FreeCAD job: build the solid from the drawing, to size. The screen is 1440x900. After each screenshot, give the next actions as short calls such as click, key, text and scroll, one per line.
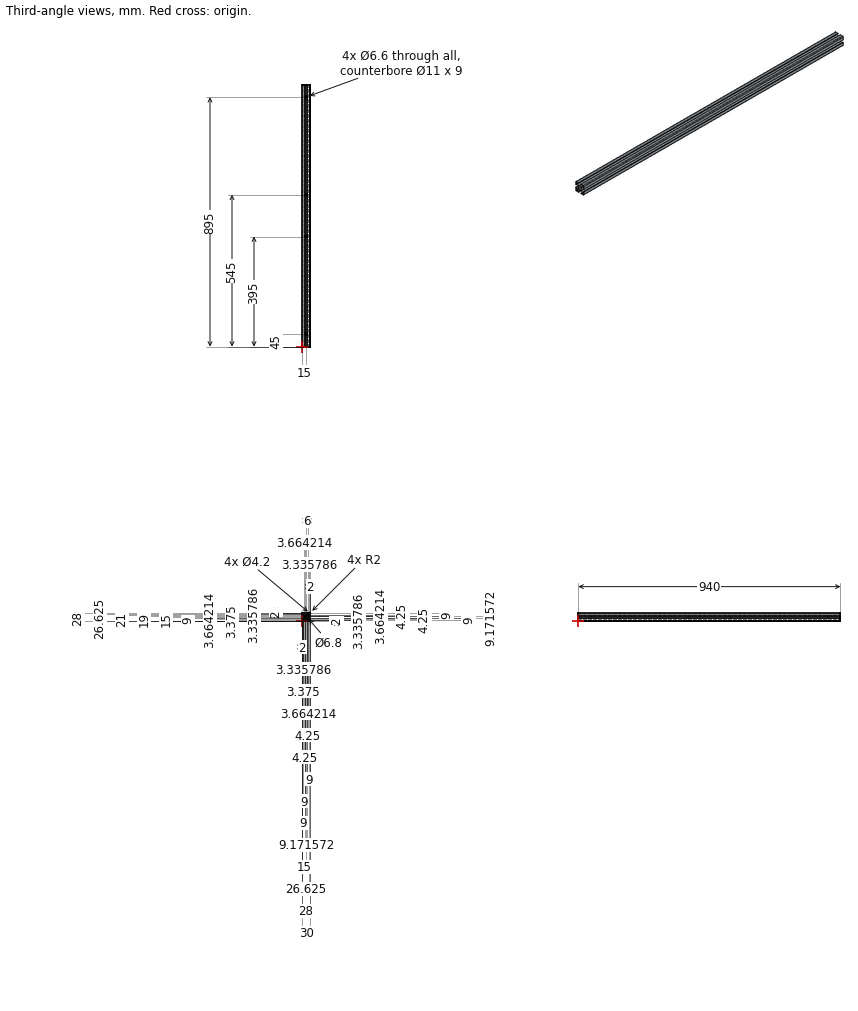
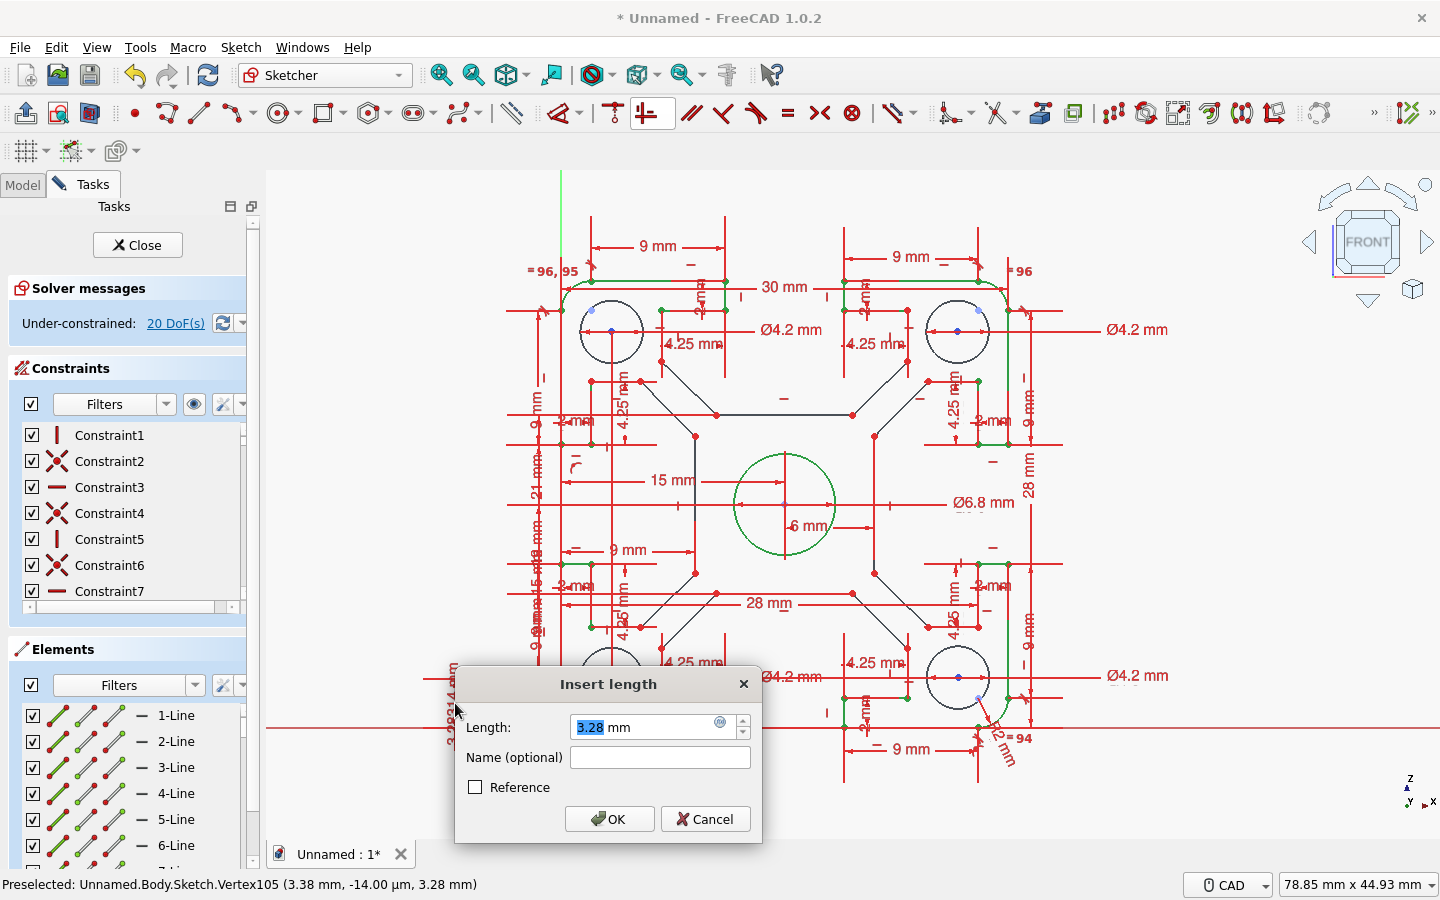
text(3.375)
key(Return)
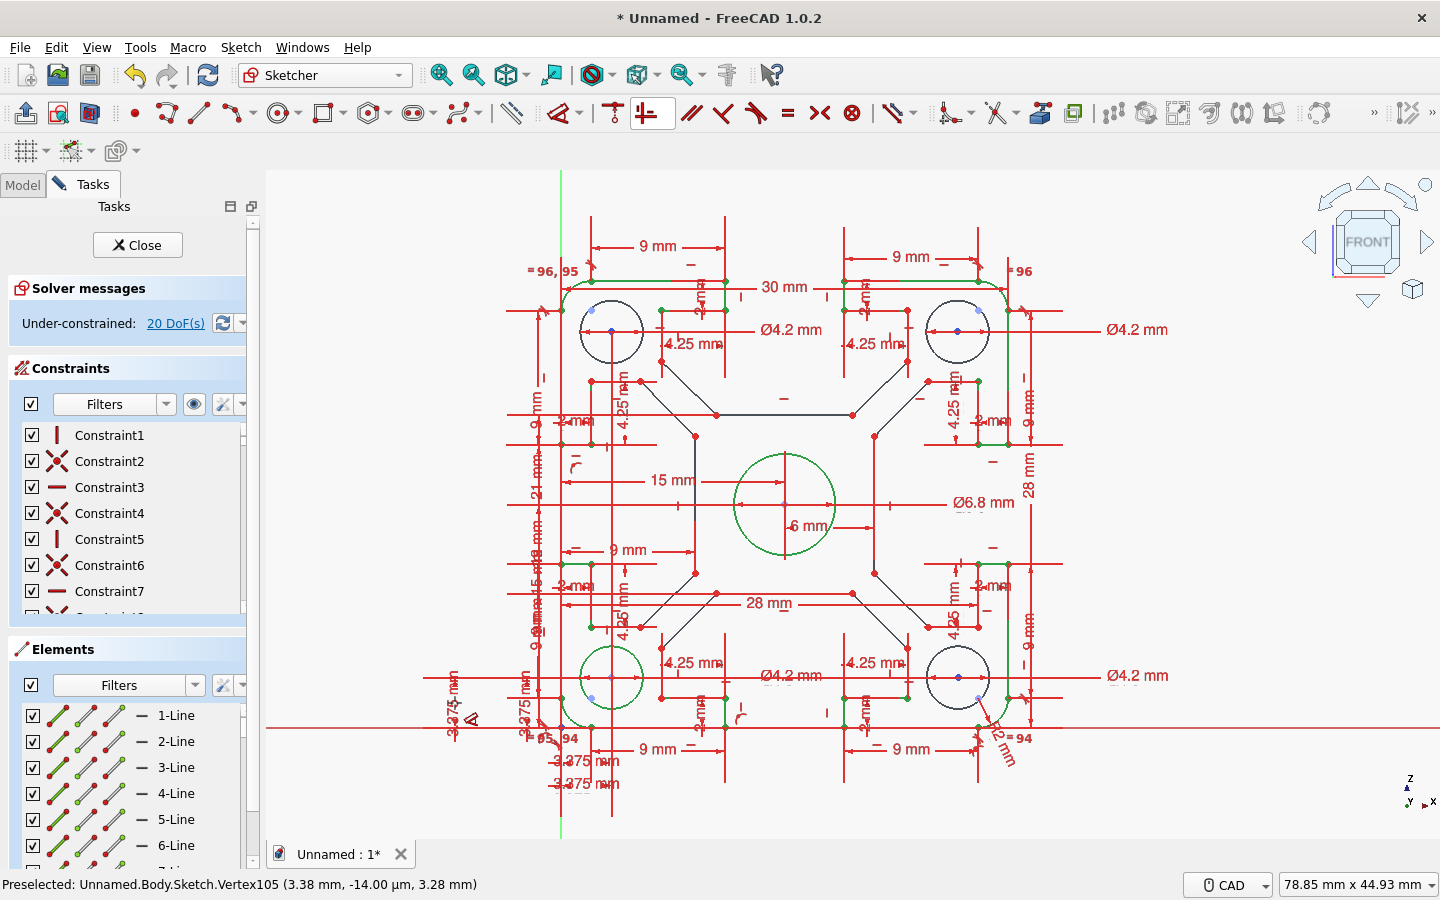
click(958, 332)
click(759, 762)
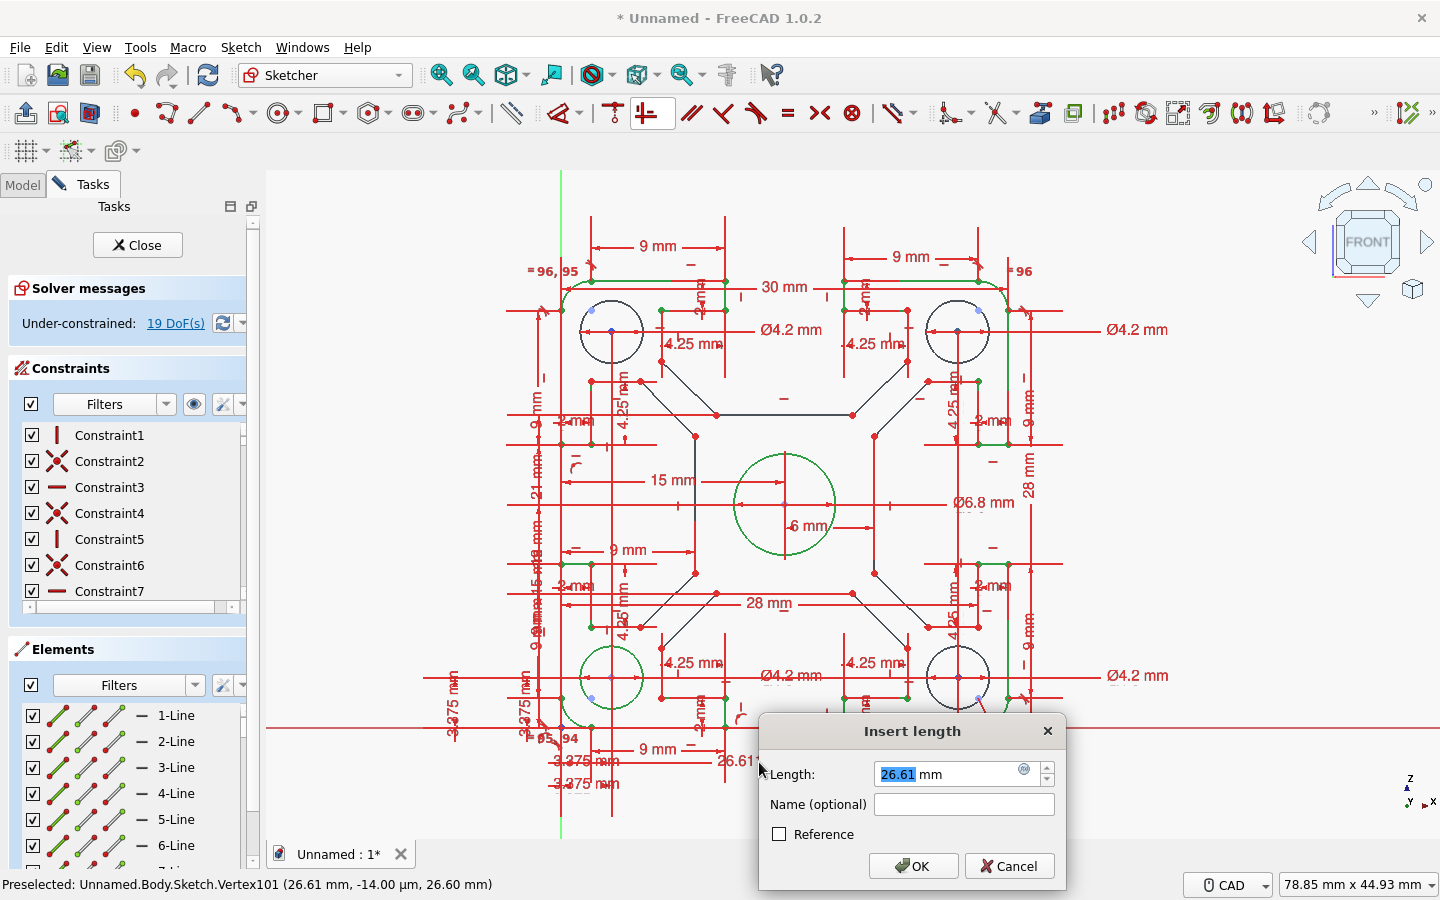
text(26.625)
key(Return)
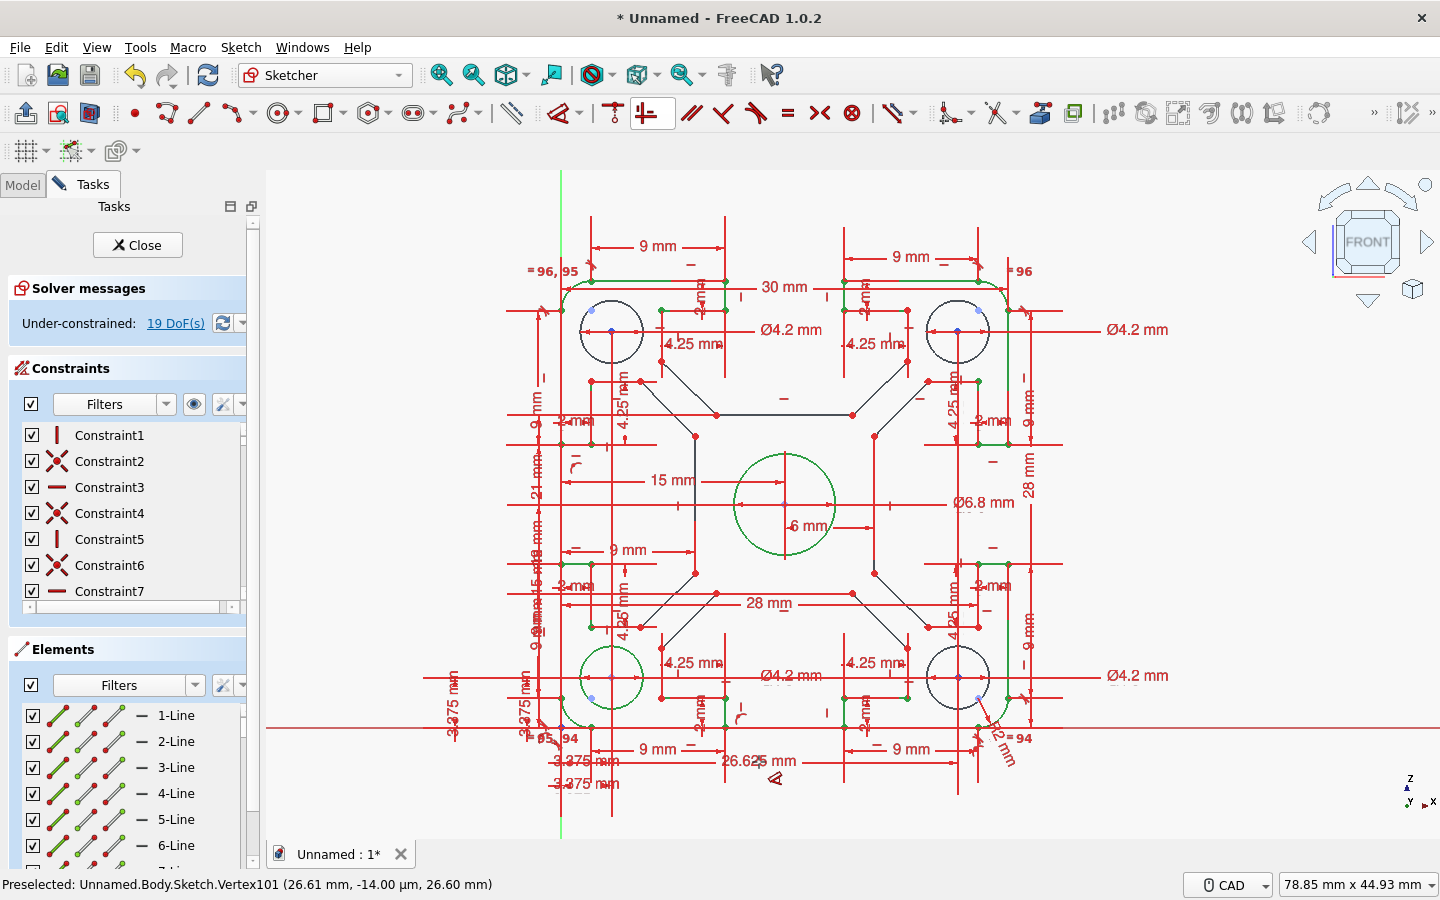
click(958, 332)
click(527, 668)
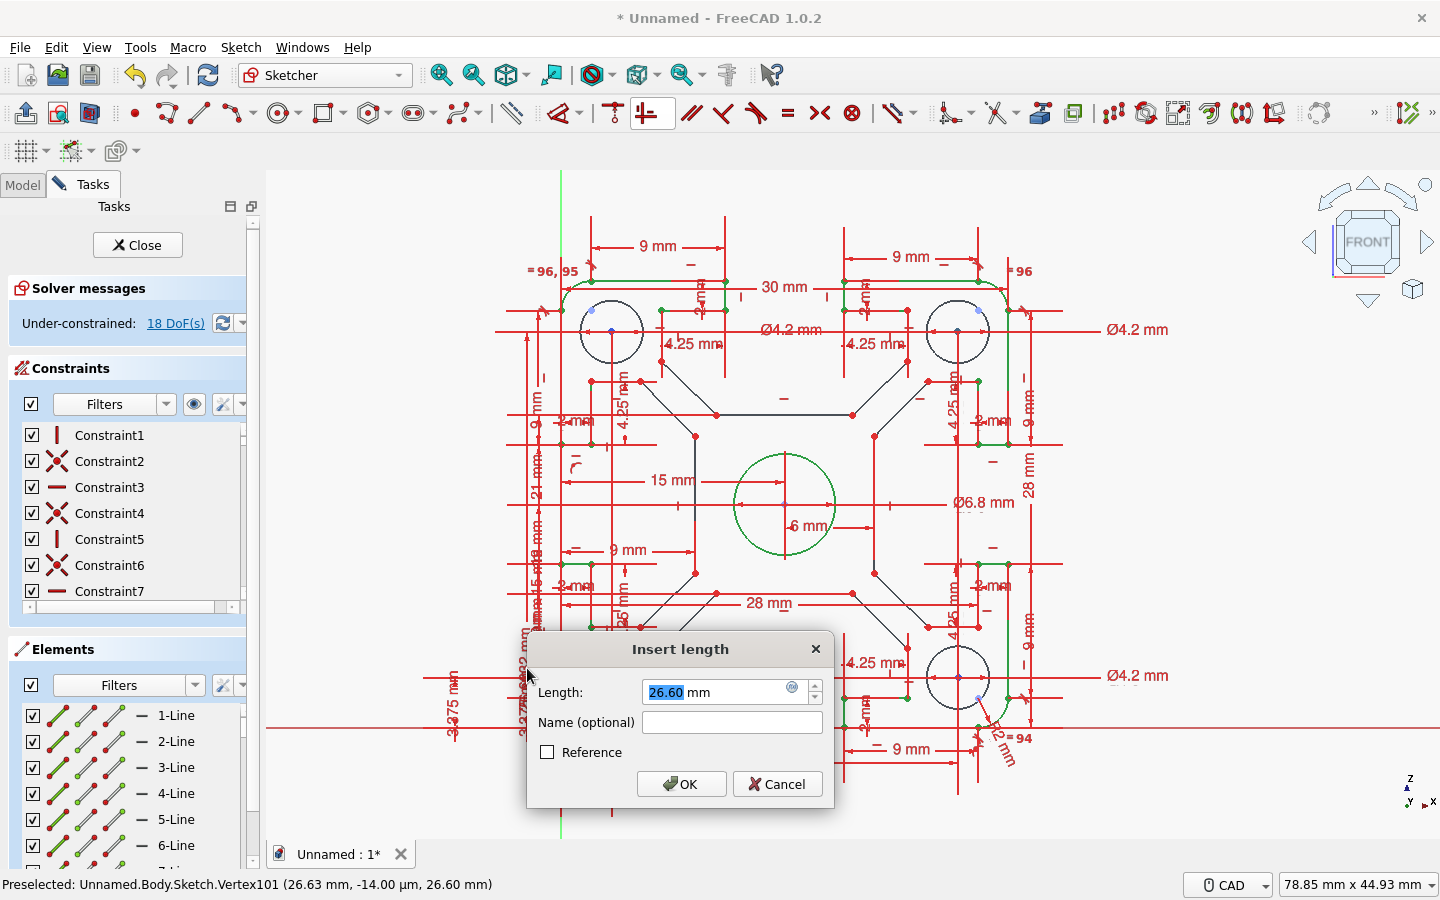
text(26.625)
key(Return)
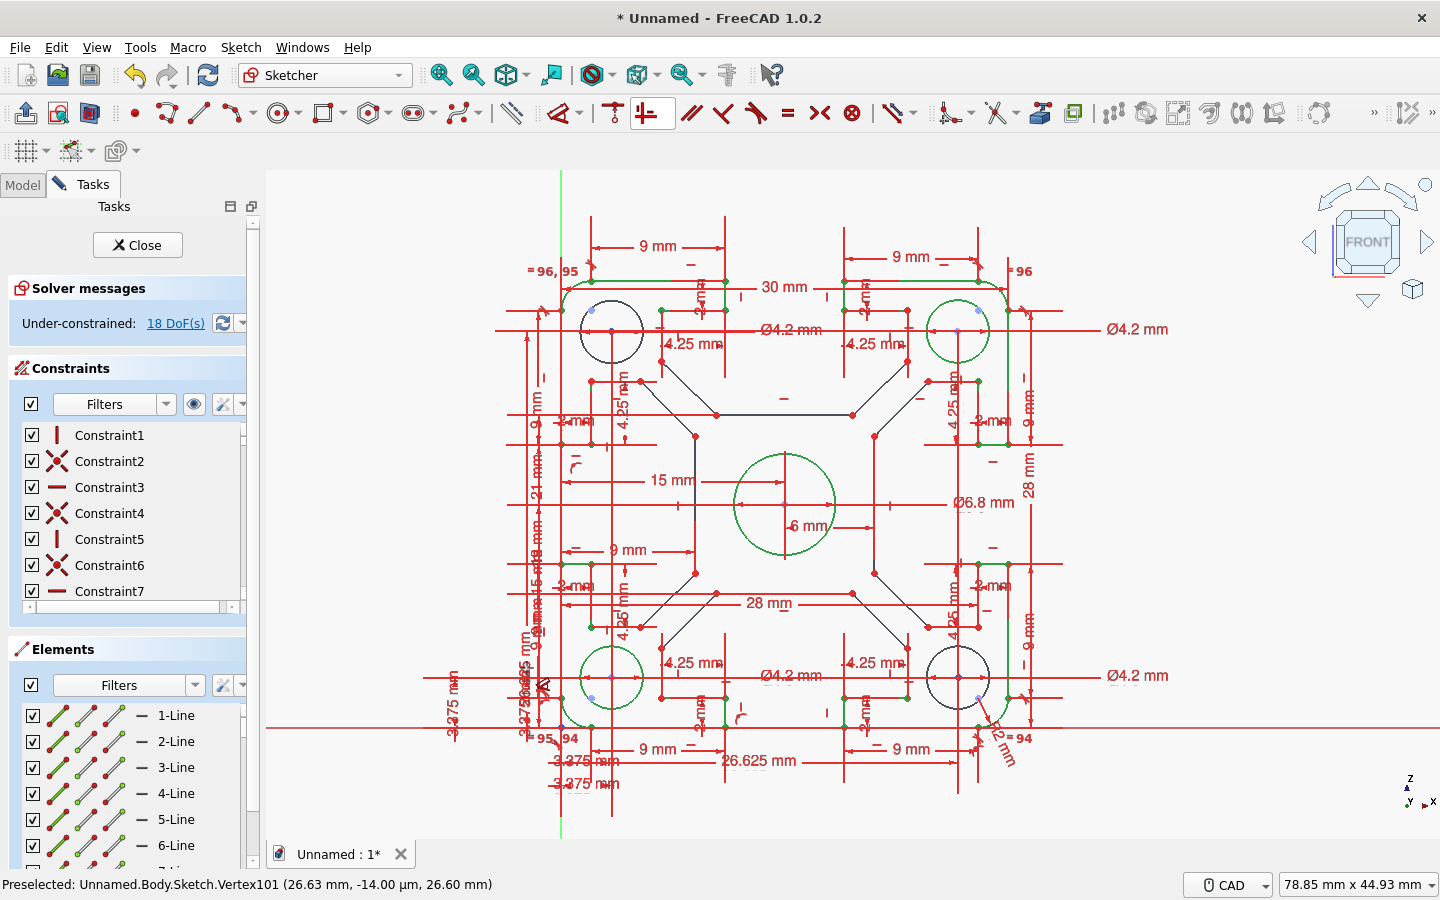
click(612, 332)
click(646, 530)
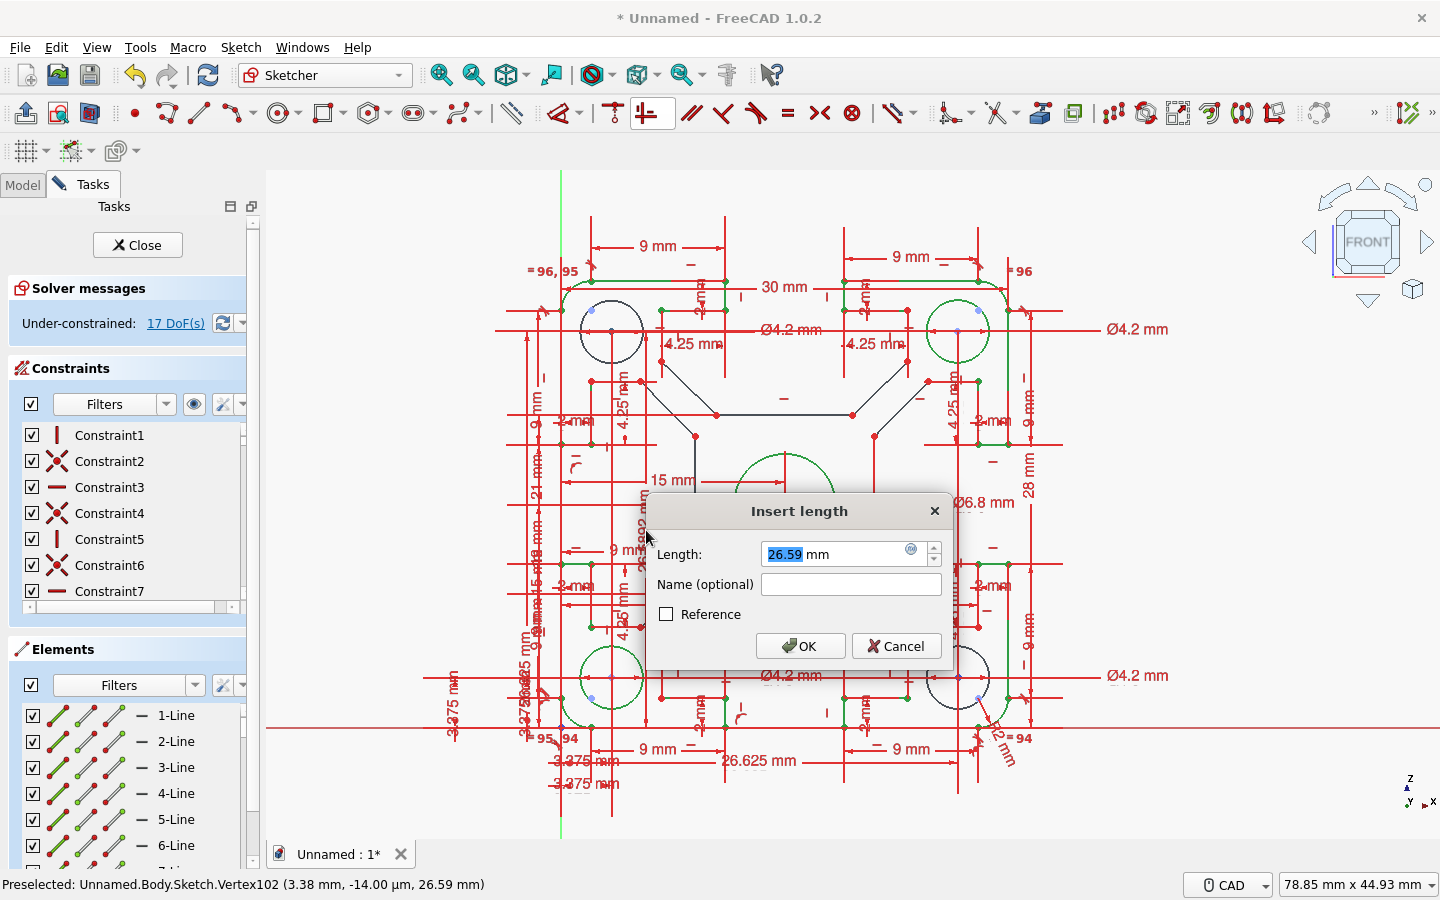
text(26.625)
key(Return)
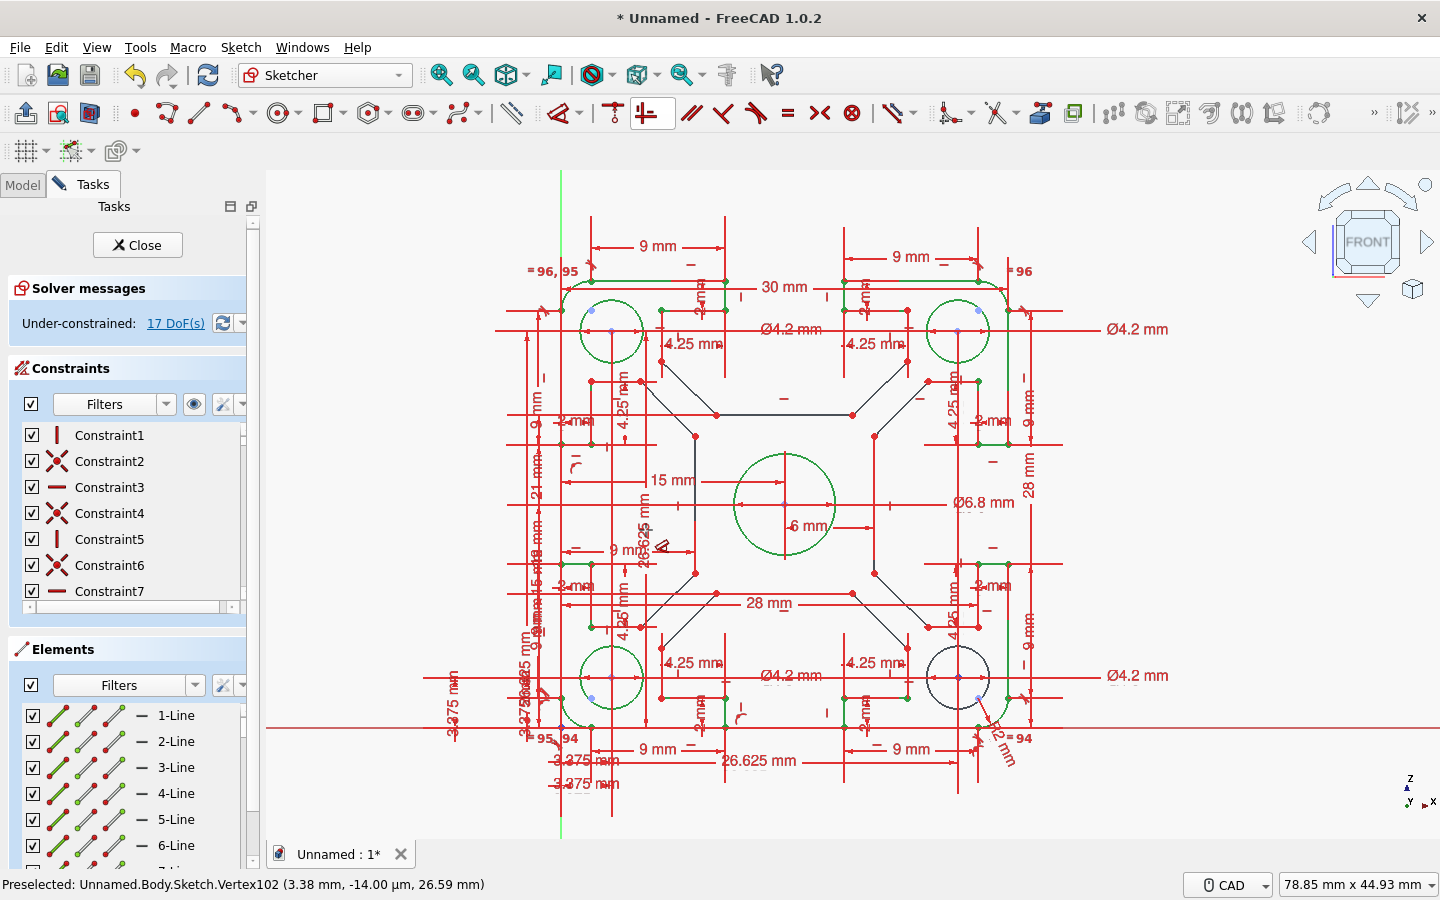
click(958, 678)
click(760, 644)